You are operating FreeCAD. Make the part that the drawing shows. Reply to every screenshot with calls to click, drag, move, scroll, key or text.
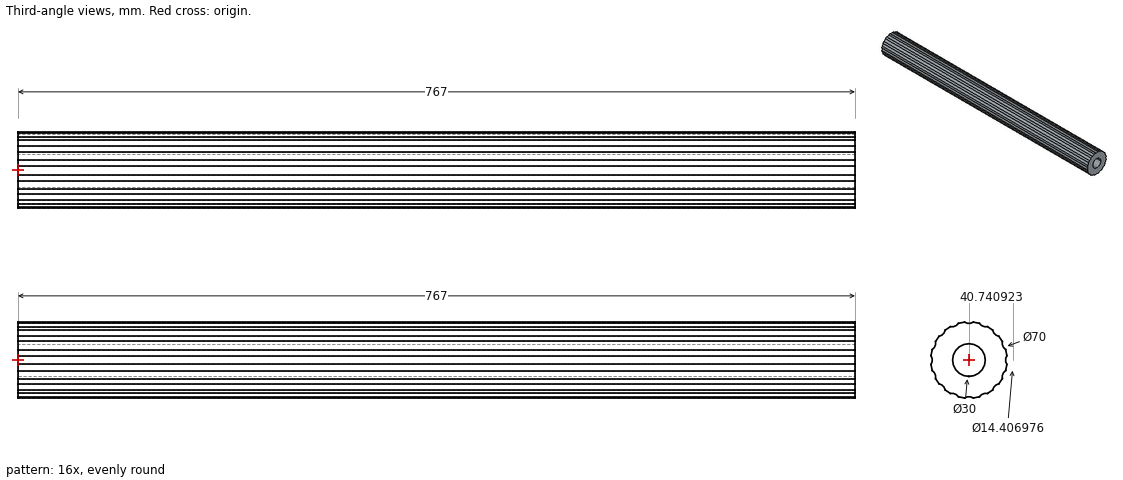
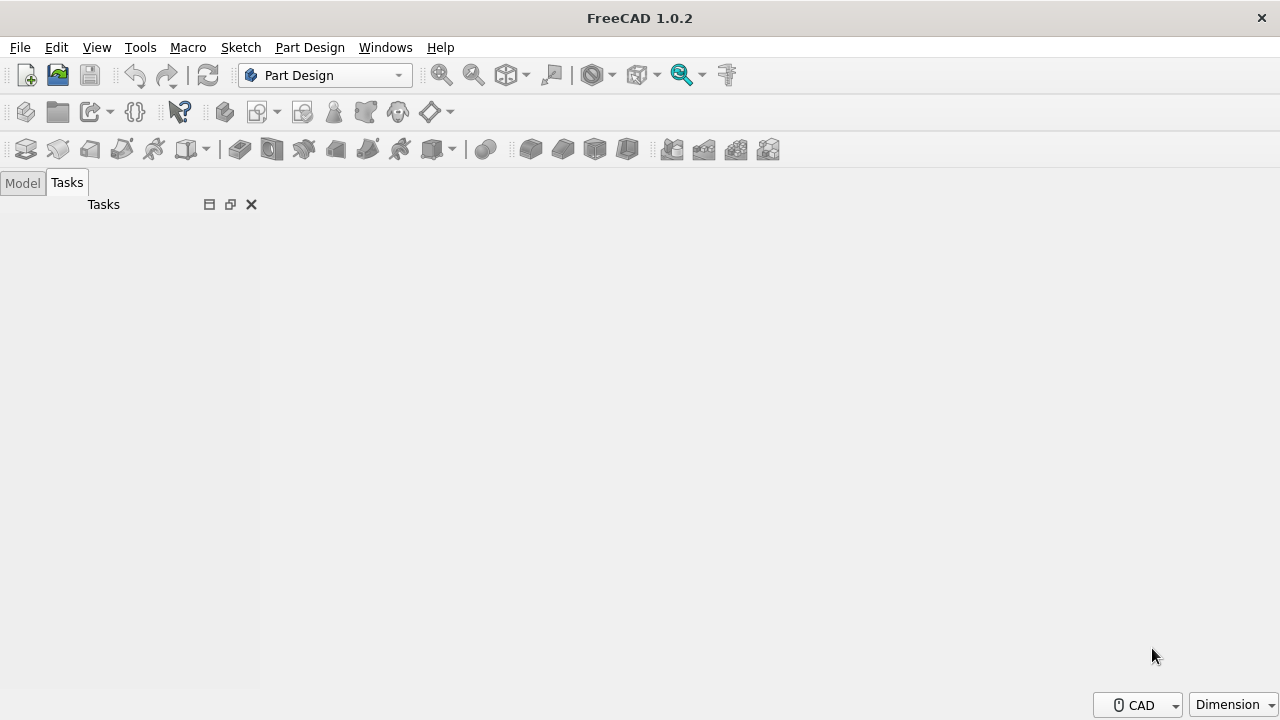
click(26, 76)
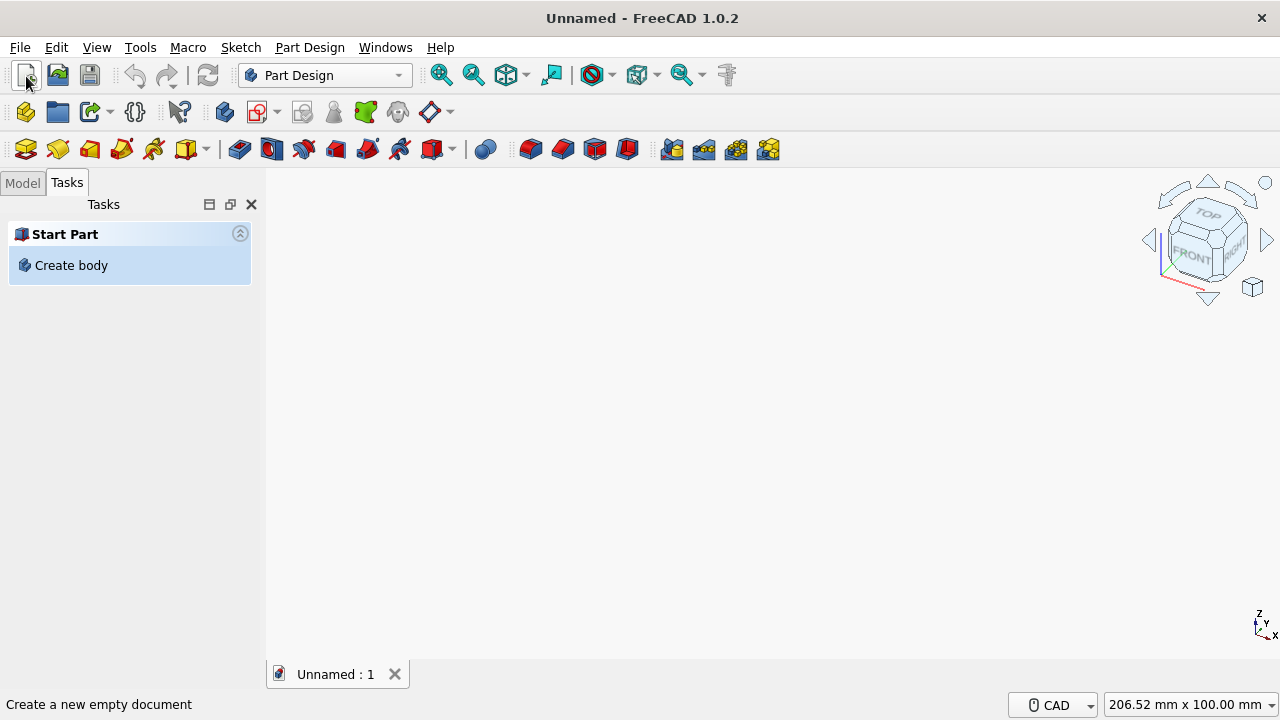
click(258, 112)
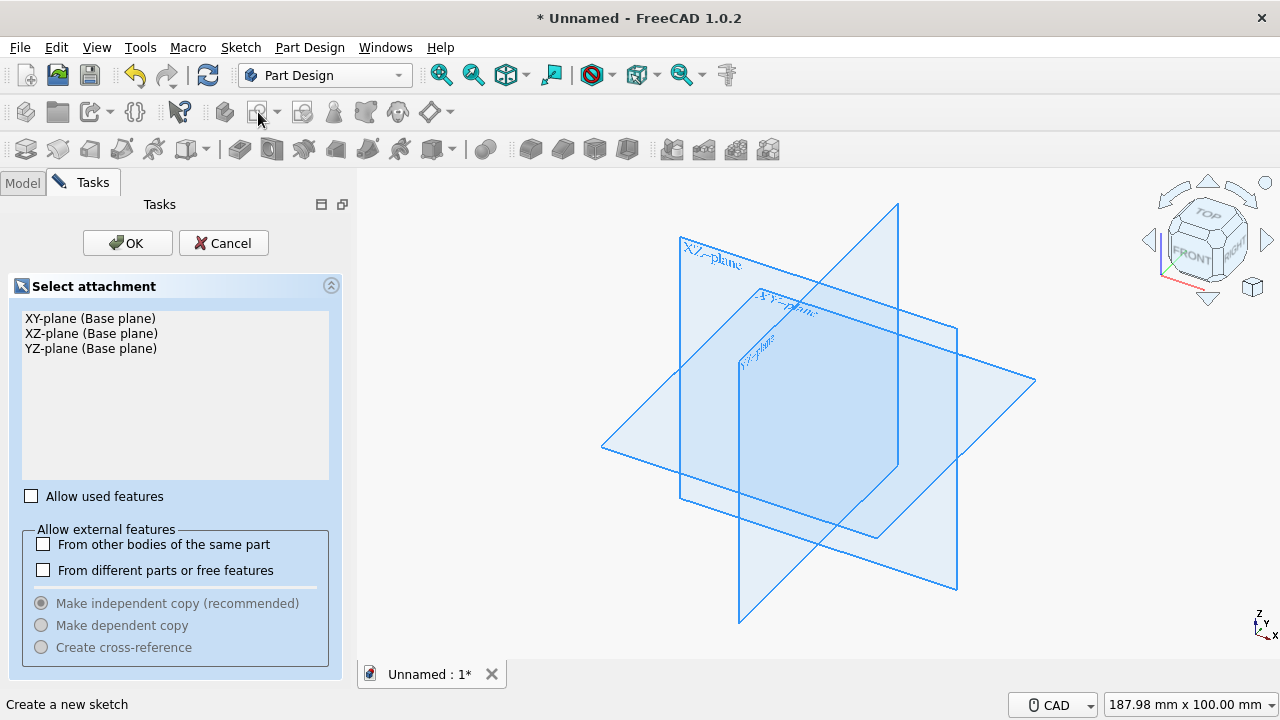
click(82, 348)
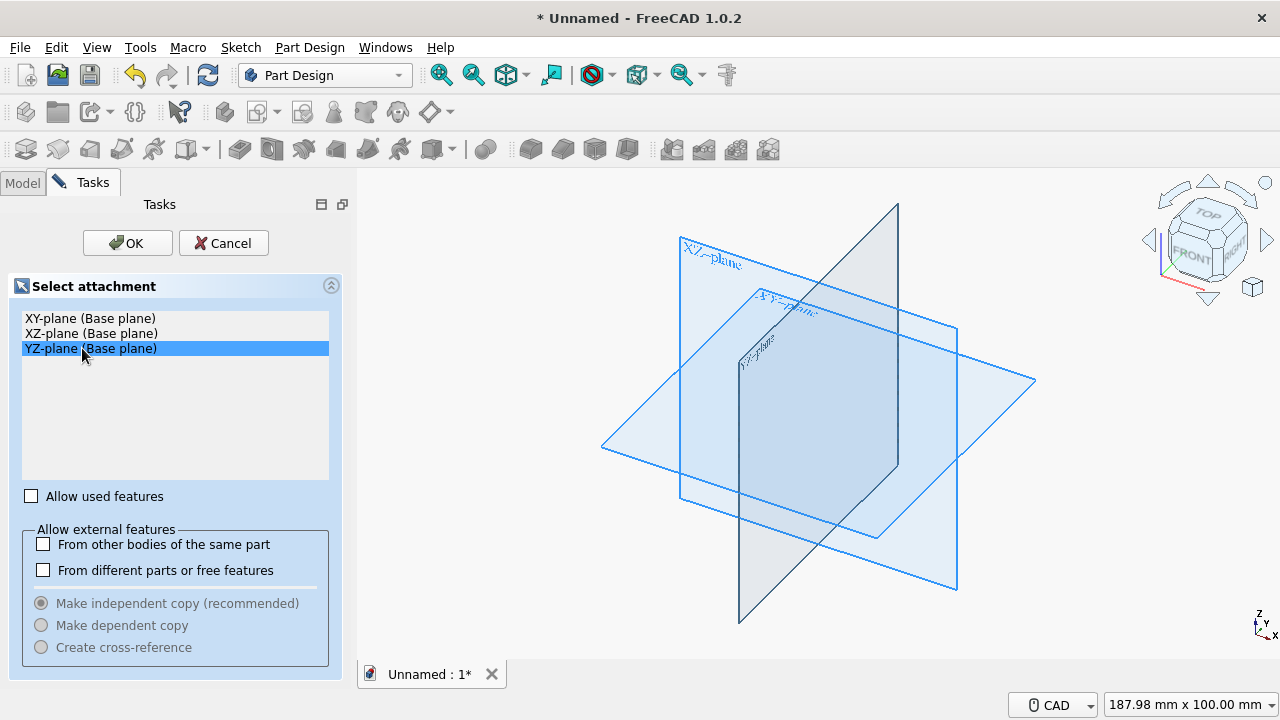
click(128, 243)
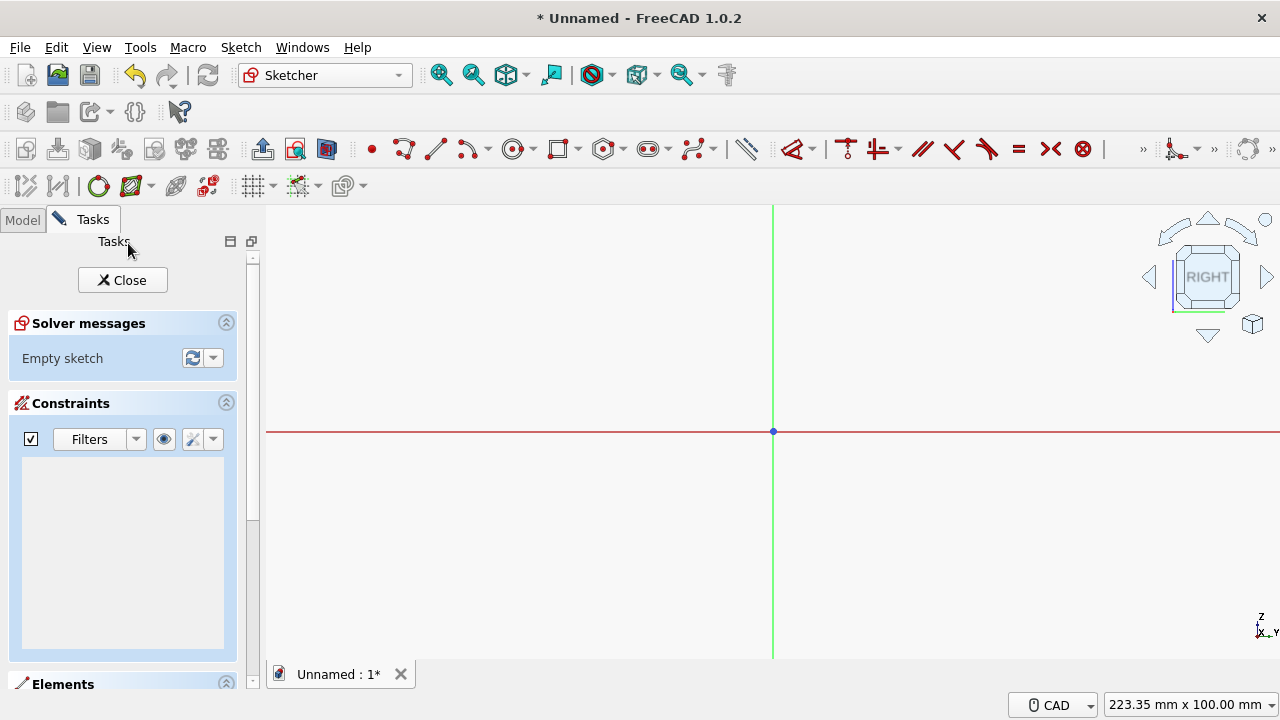
click(514, 150)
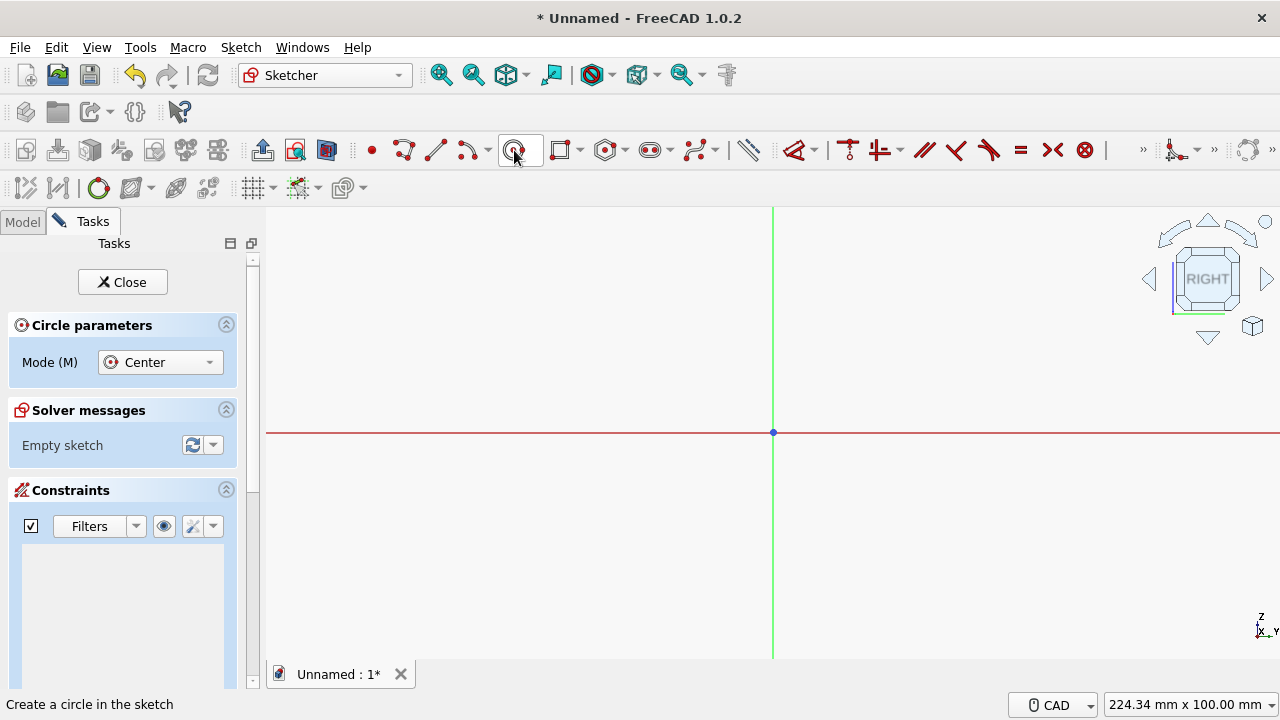
click(773, 433)
click(885, 321)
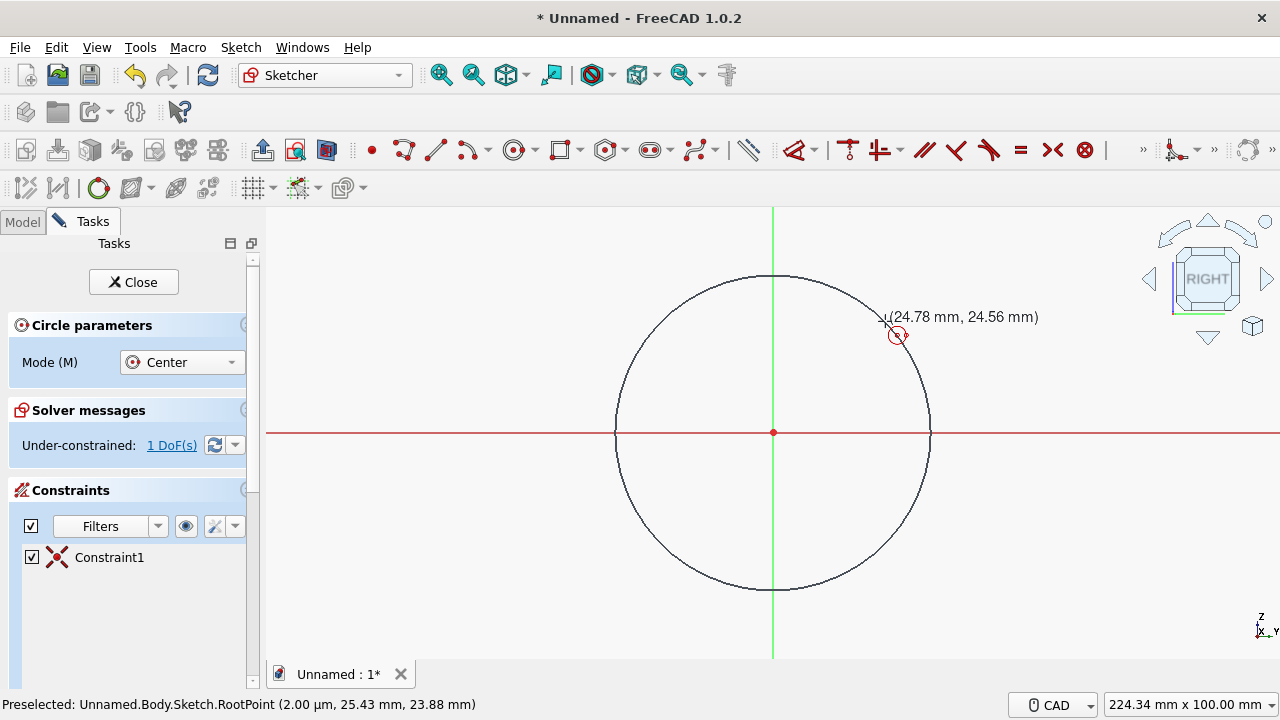
click(773, 433)
click(821, 385)
key(Escape)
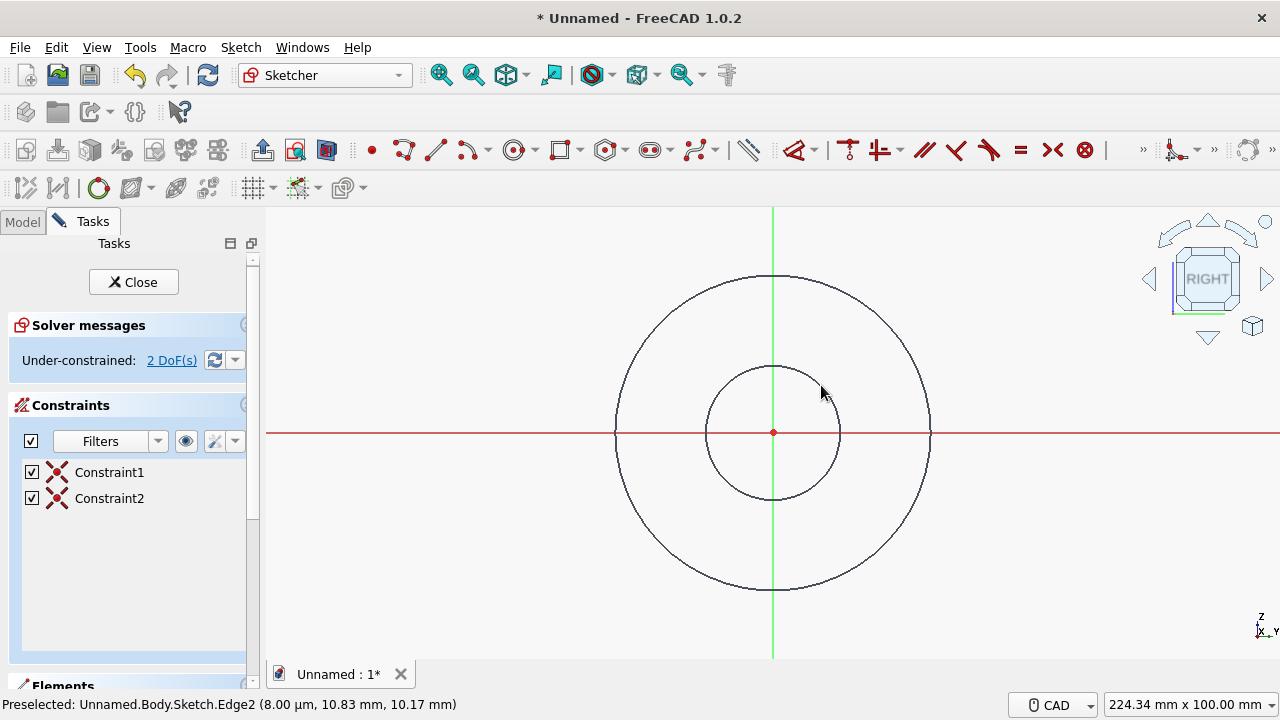
click(884, 321)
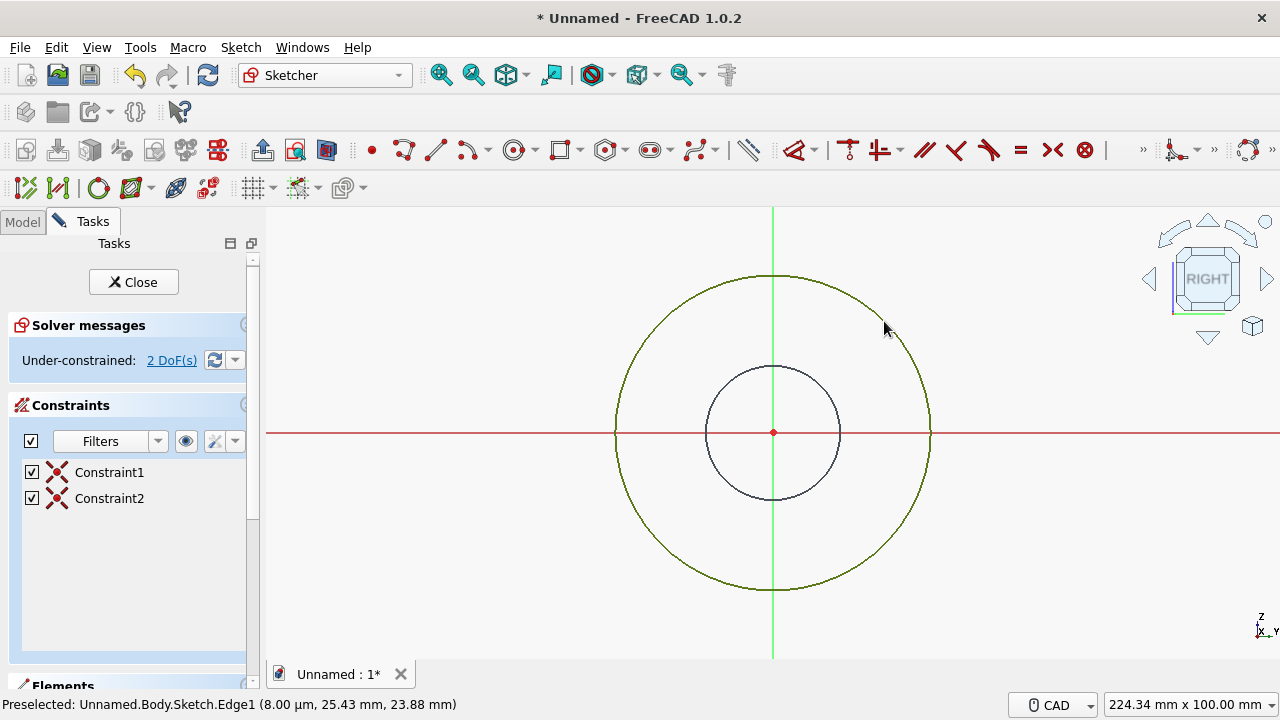
click(816, 150)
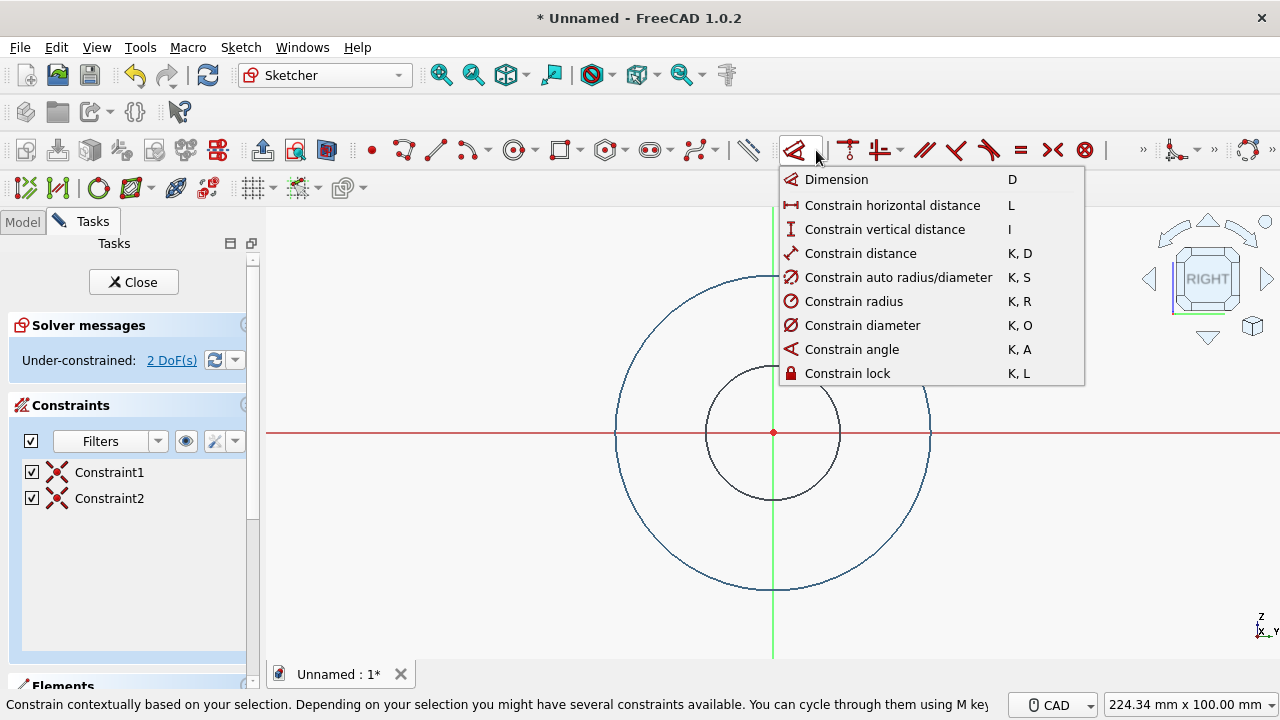
click(932, 325)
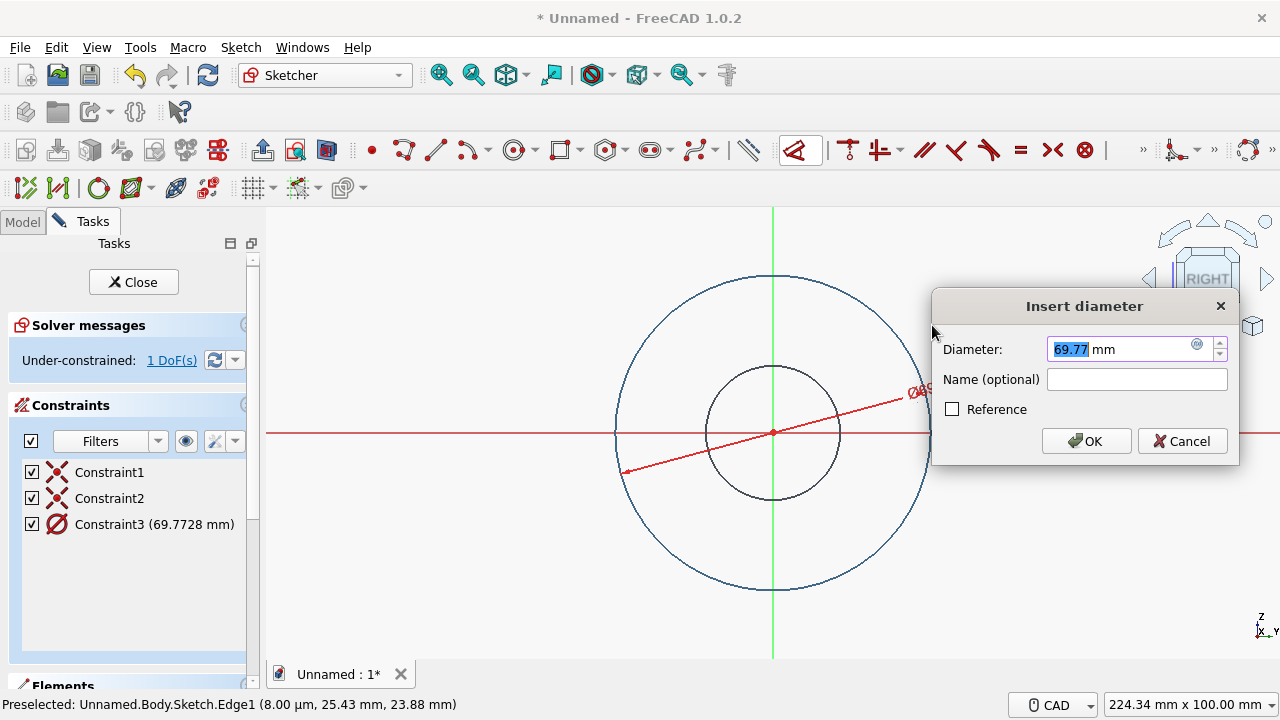
text(70)
key(Return)